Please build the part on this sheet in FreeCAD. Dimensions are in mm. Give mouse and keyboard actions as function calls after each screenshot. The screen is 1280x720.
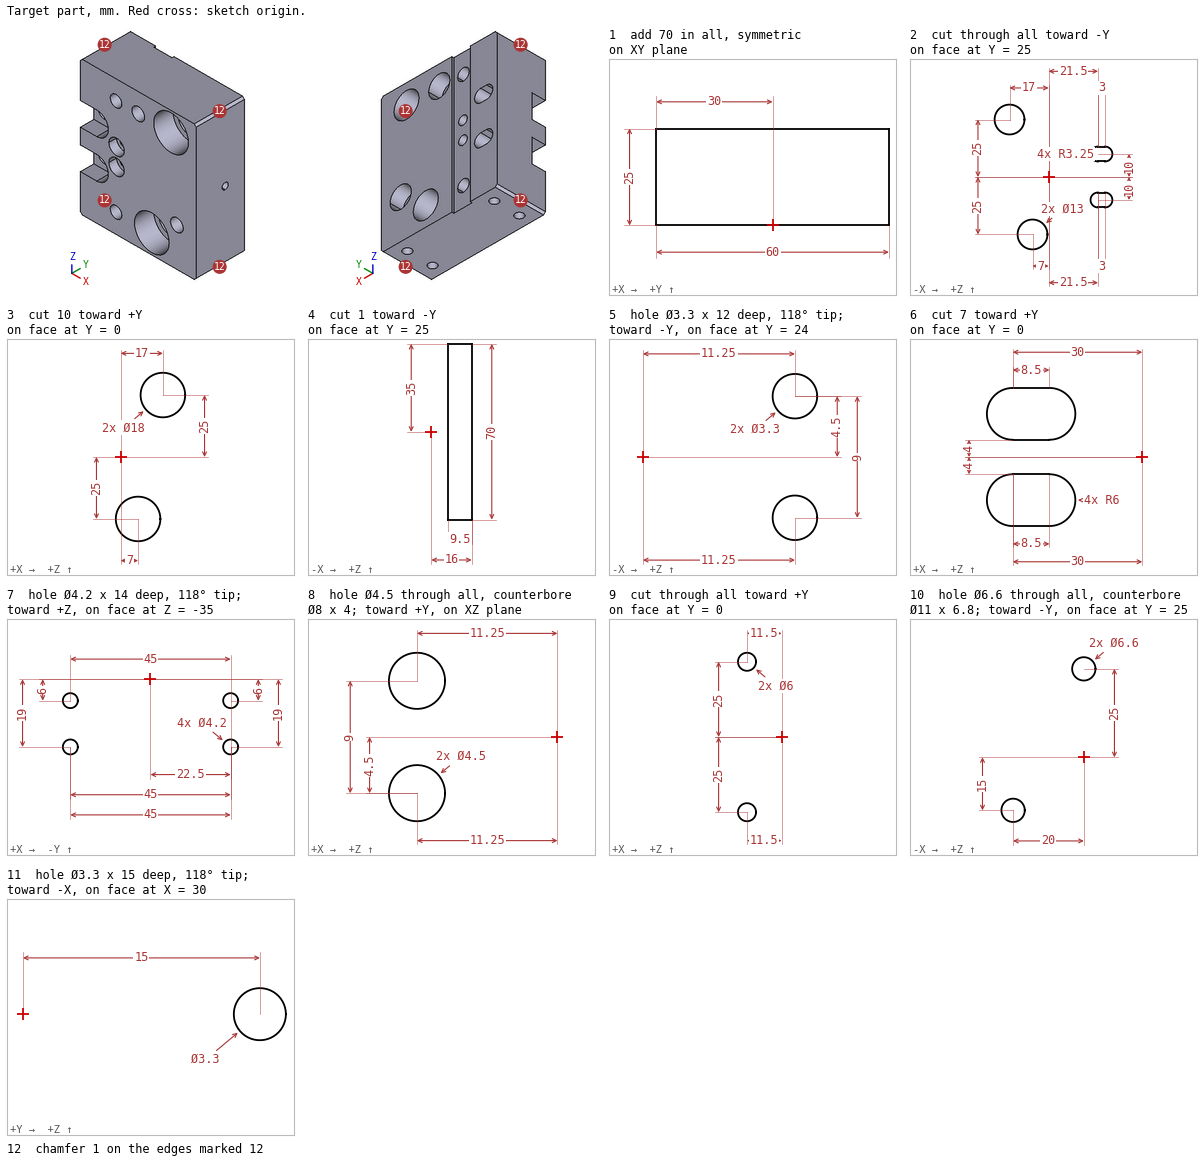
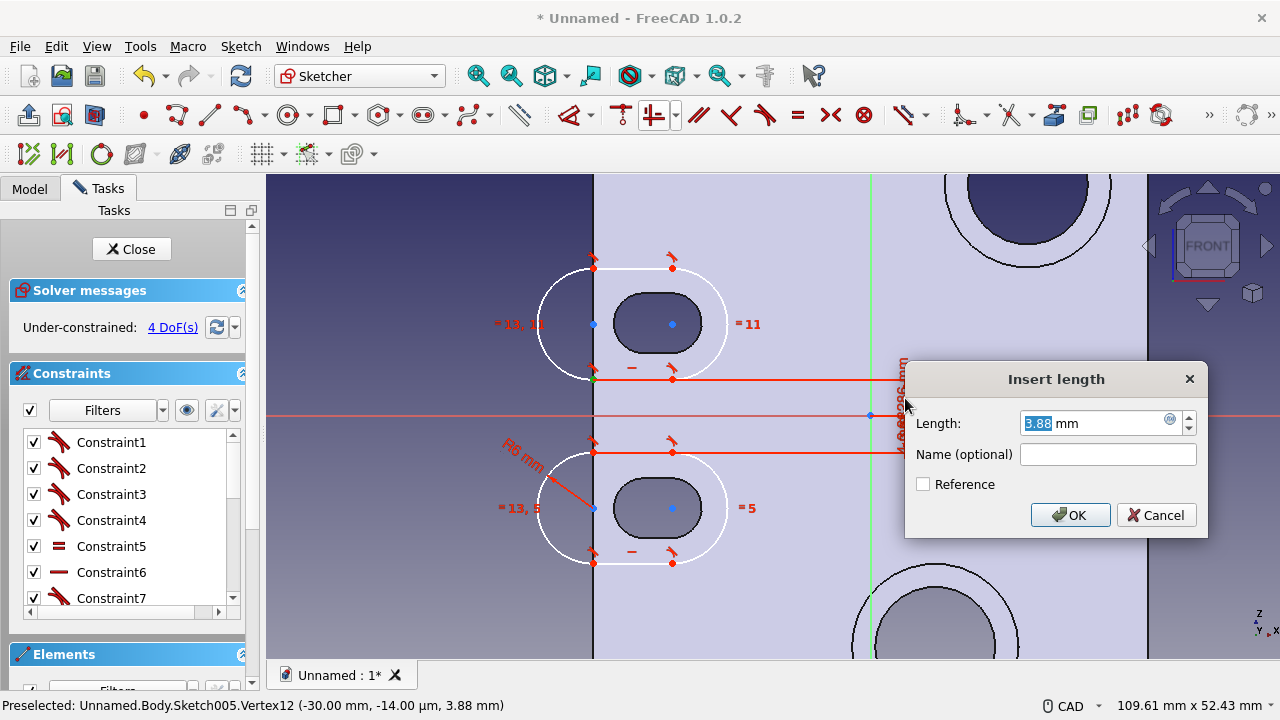
text(4)
key(Return)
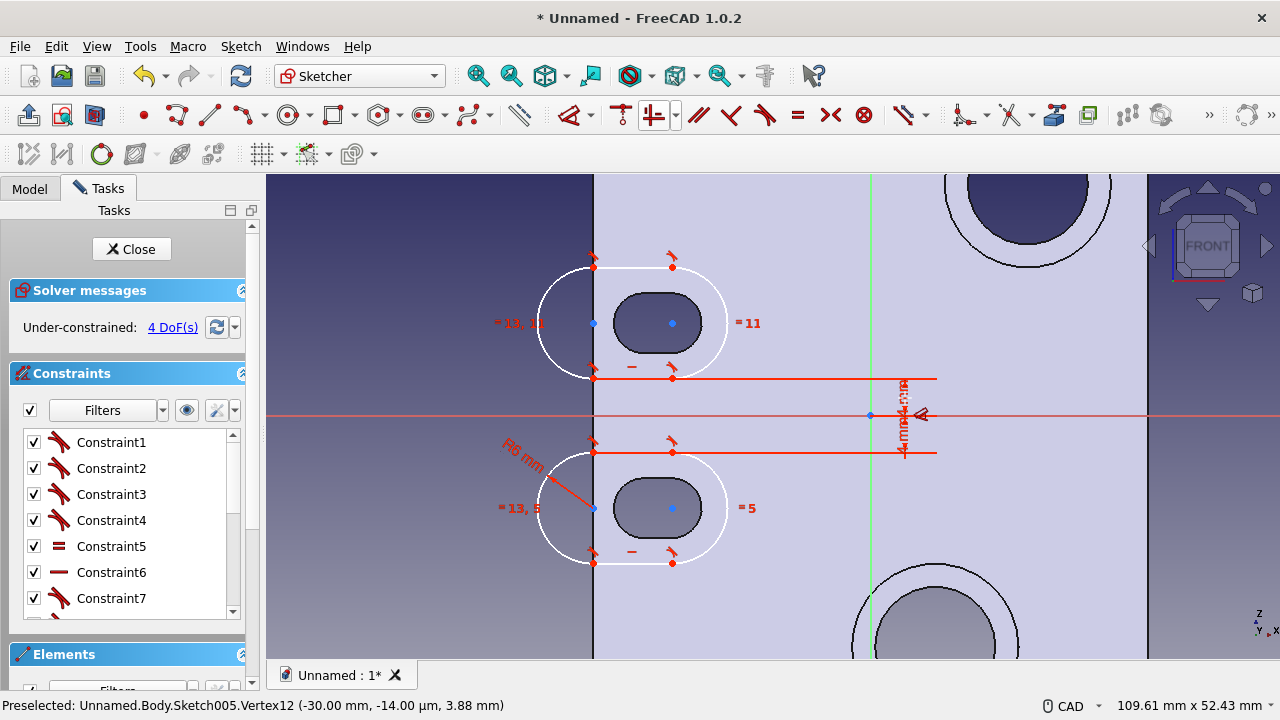
click(617, 453)
click(632, 487)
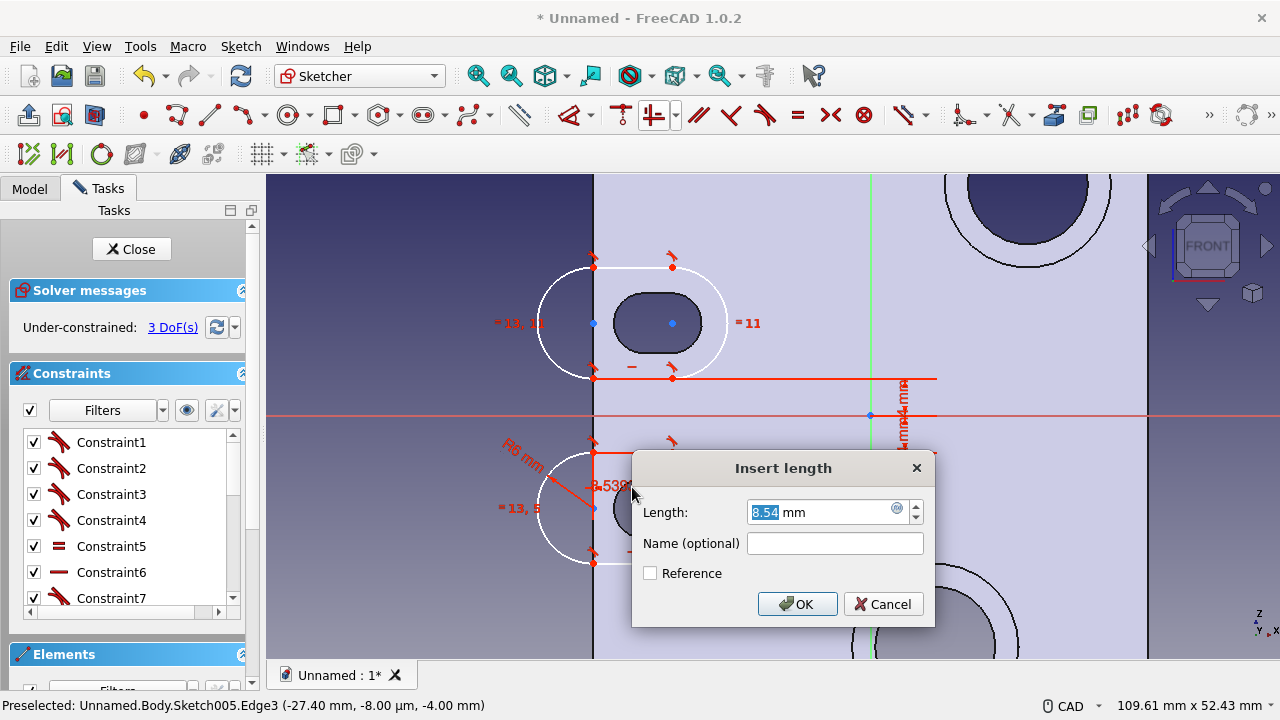
text(8.5)
key(Return)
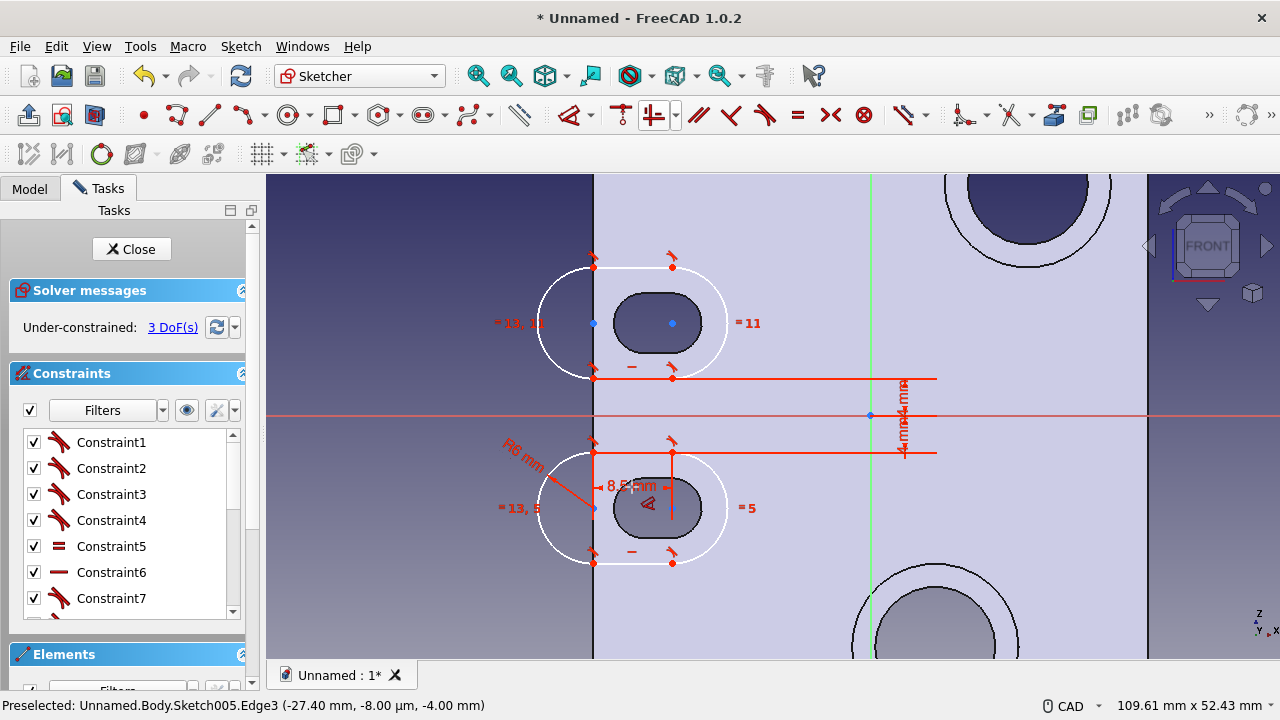
click(617, 268)
click(632, 234)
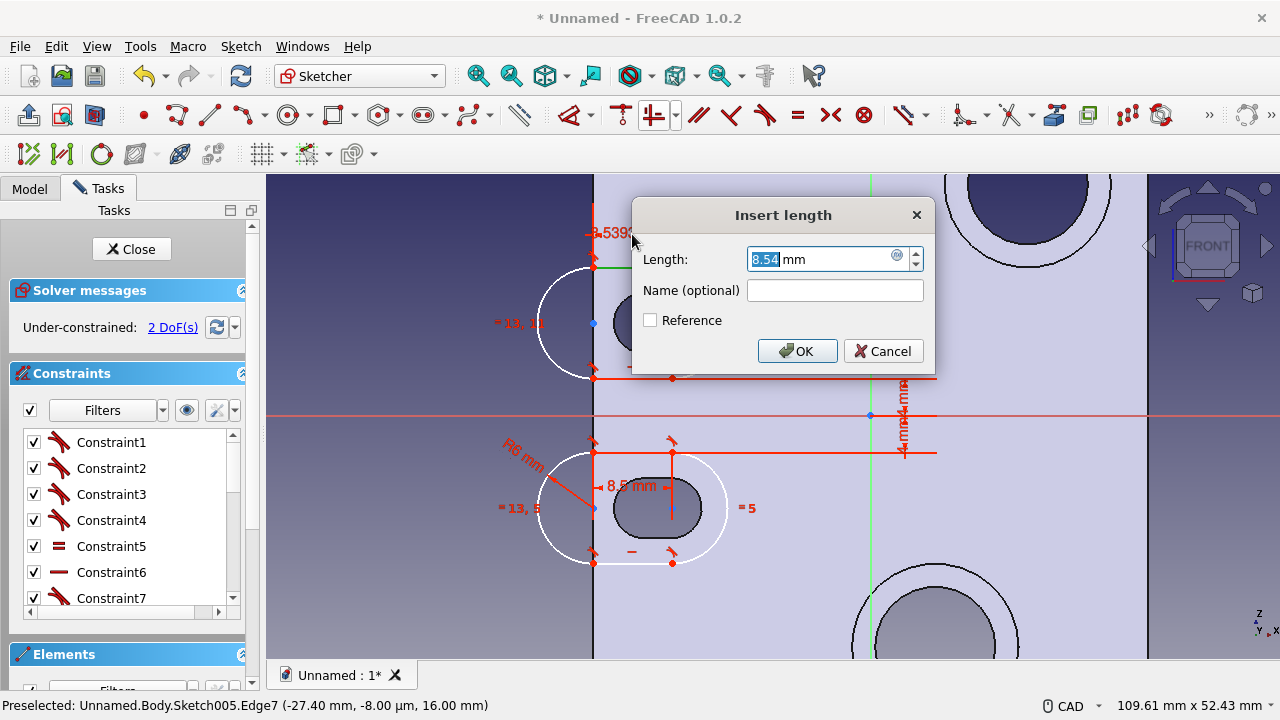
text(8.5)
key(Return)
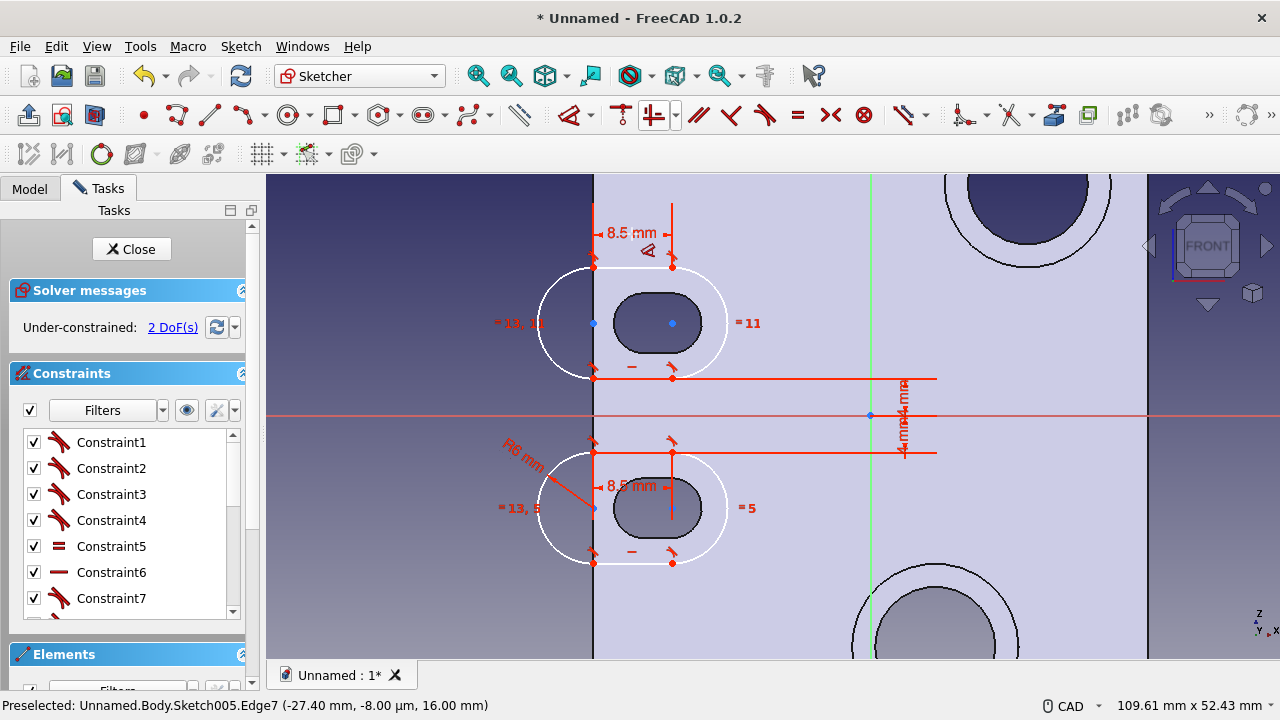
click(593, 453)
click(796, 487)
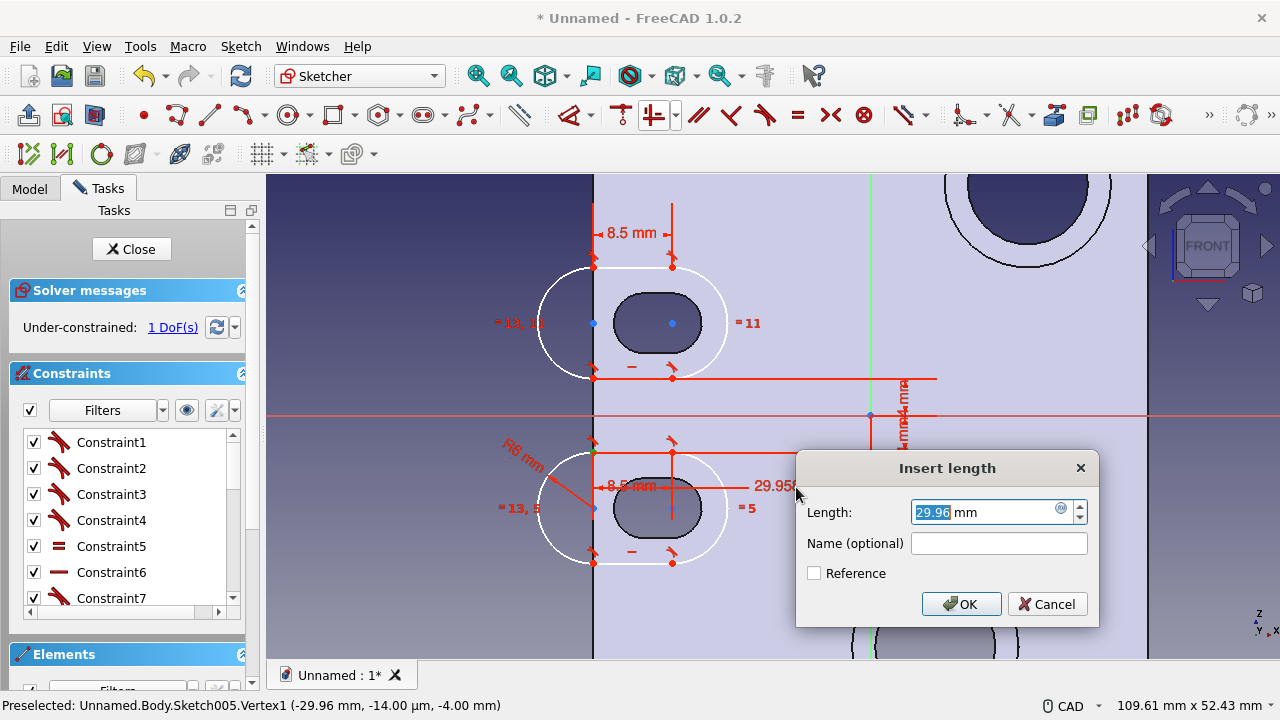
text(30)
key(Return)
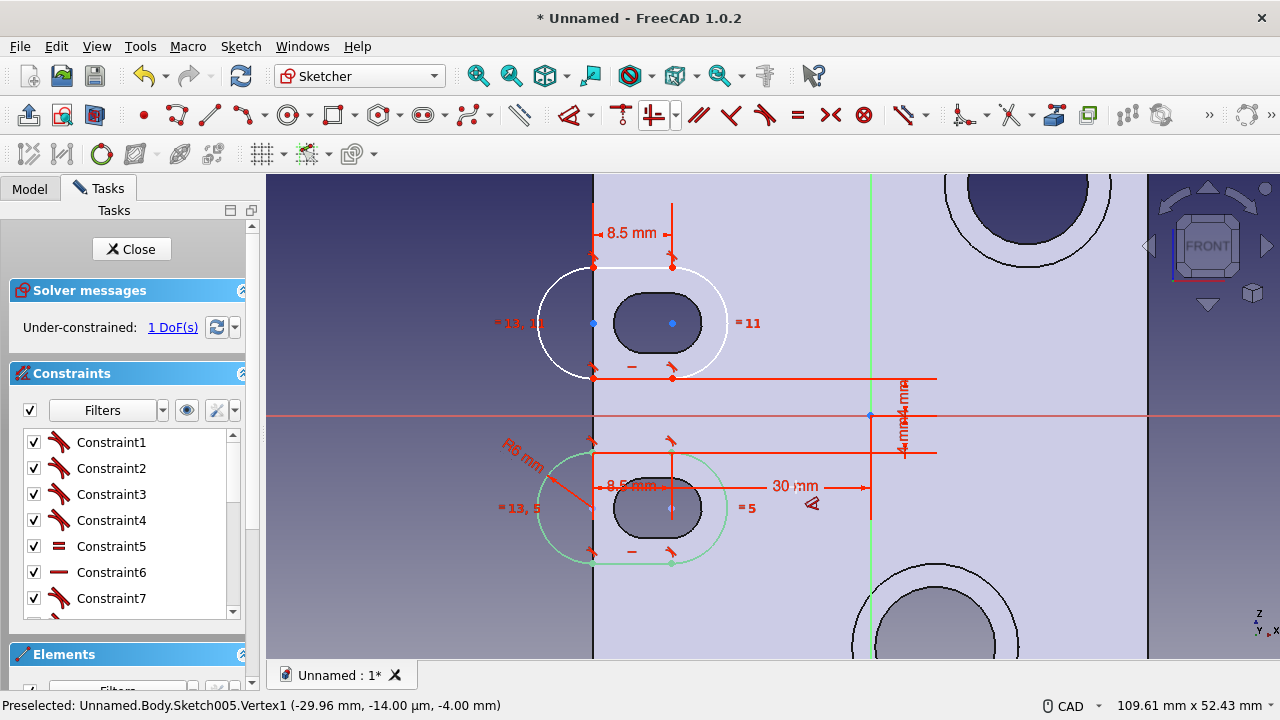
click(593, 268)
click(732, 234)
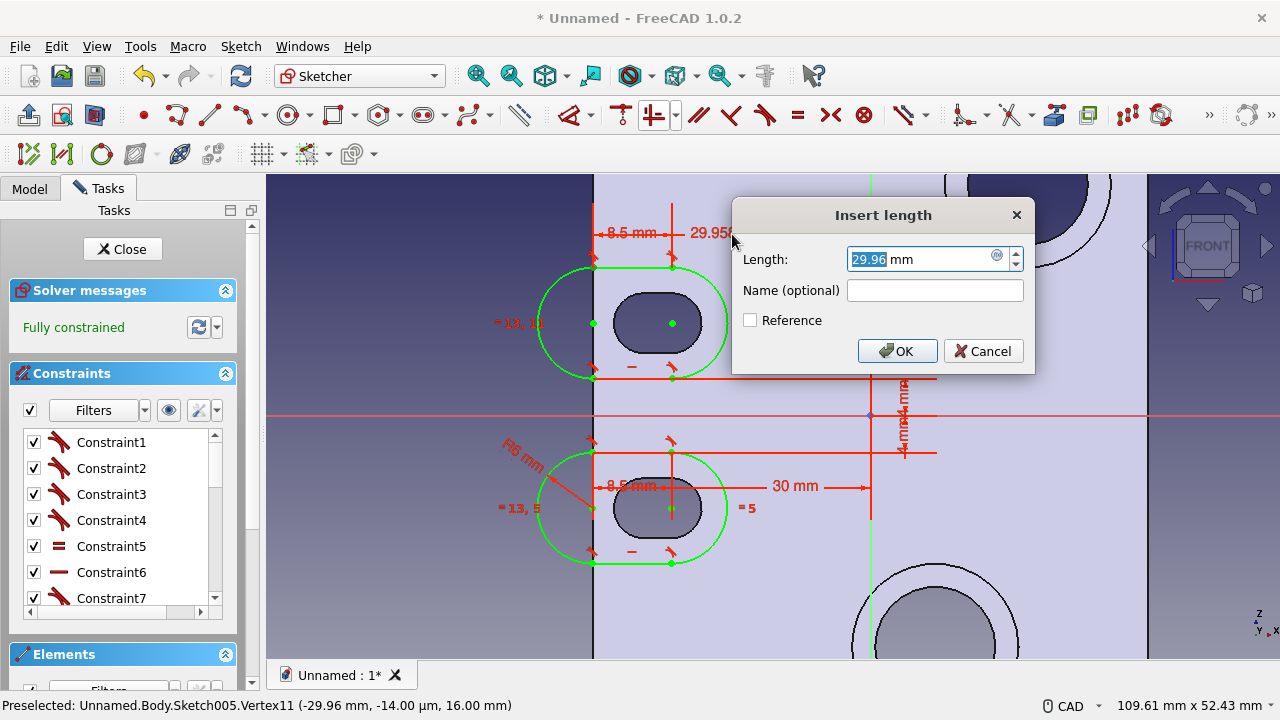
text(30)
key(Return)
key(Escape)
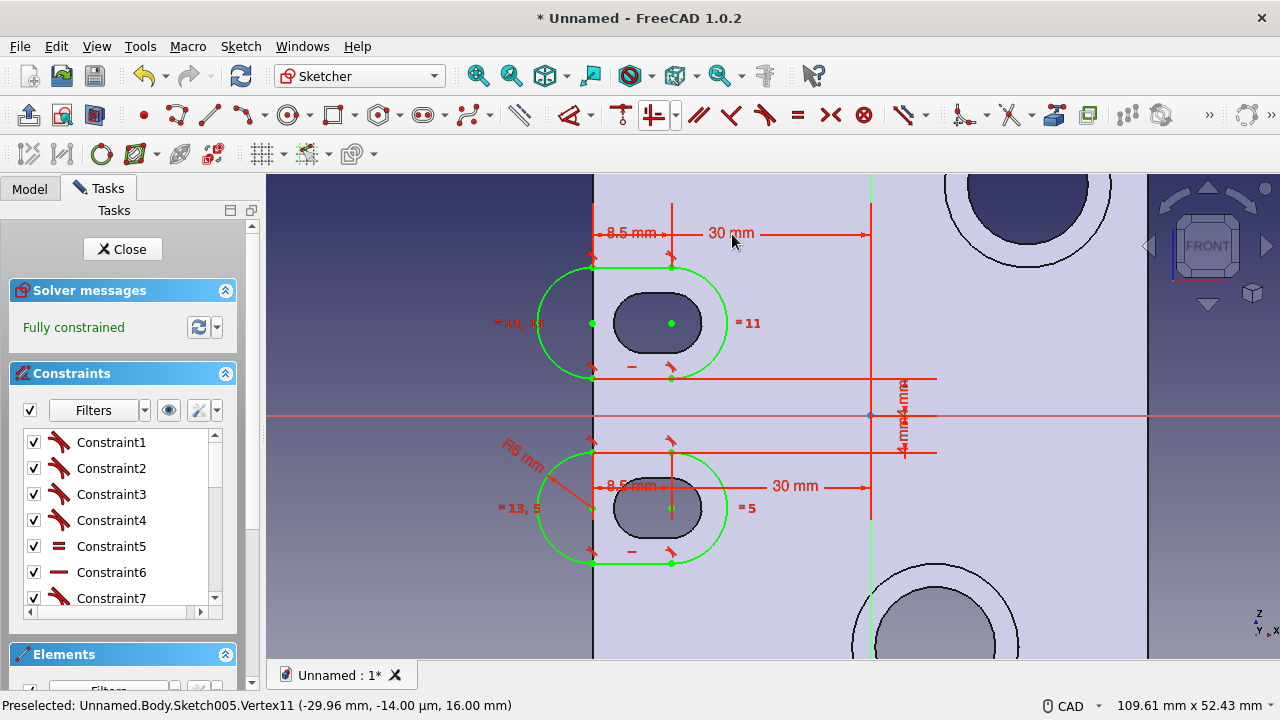
click(123, 249)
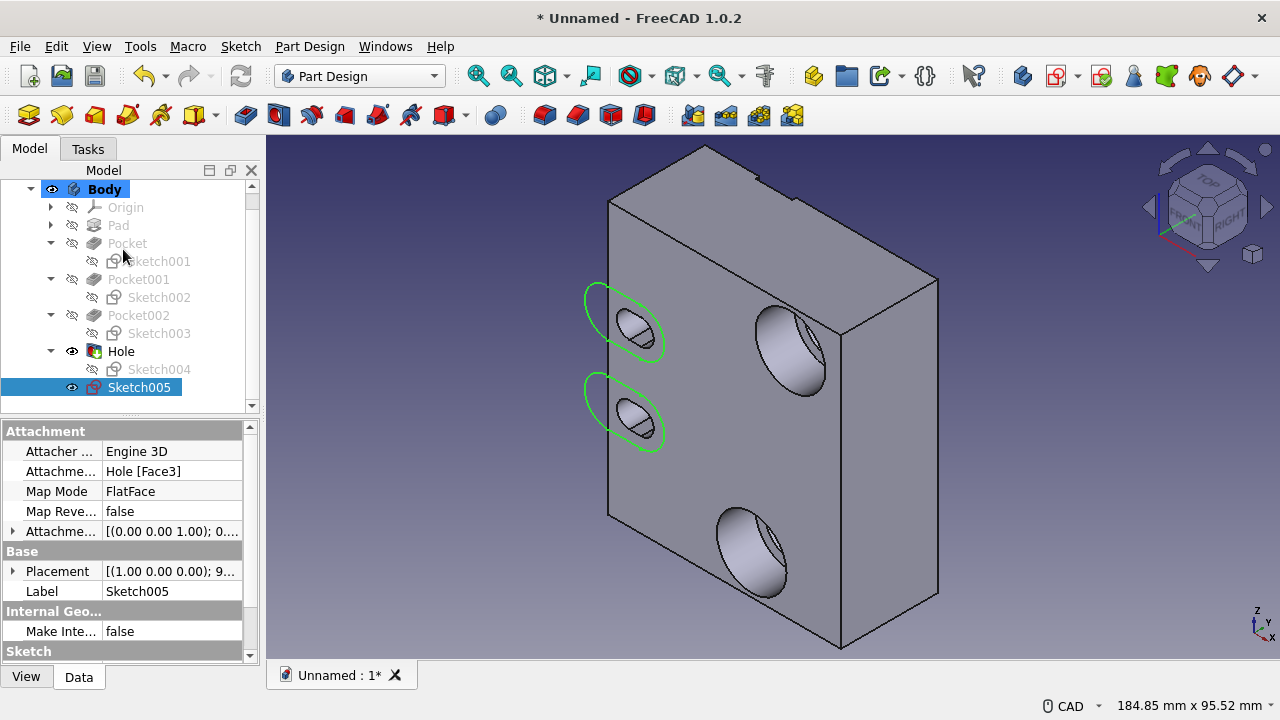
click(246, 116)